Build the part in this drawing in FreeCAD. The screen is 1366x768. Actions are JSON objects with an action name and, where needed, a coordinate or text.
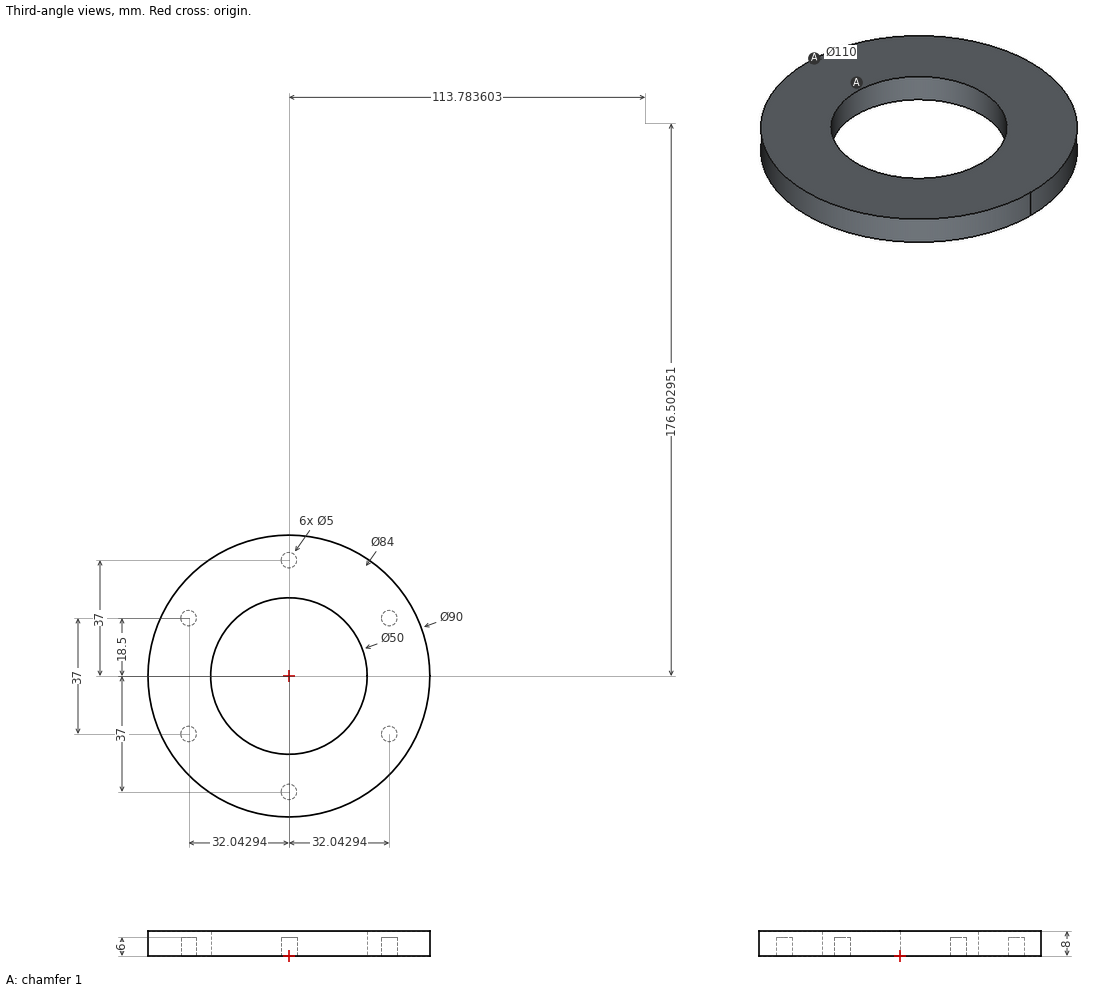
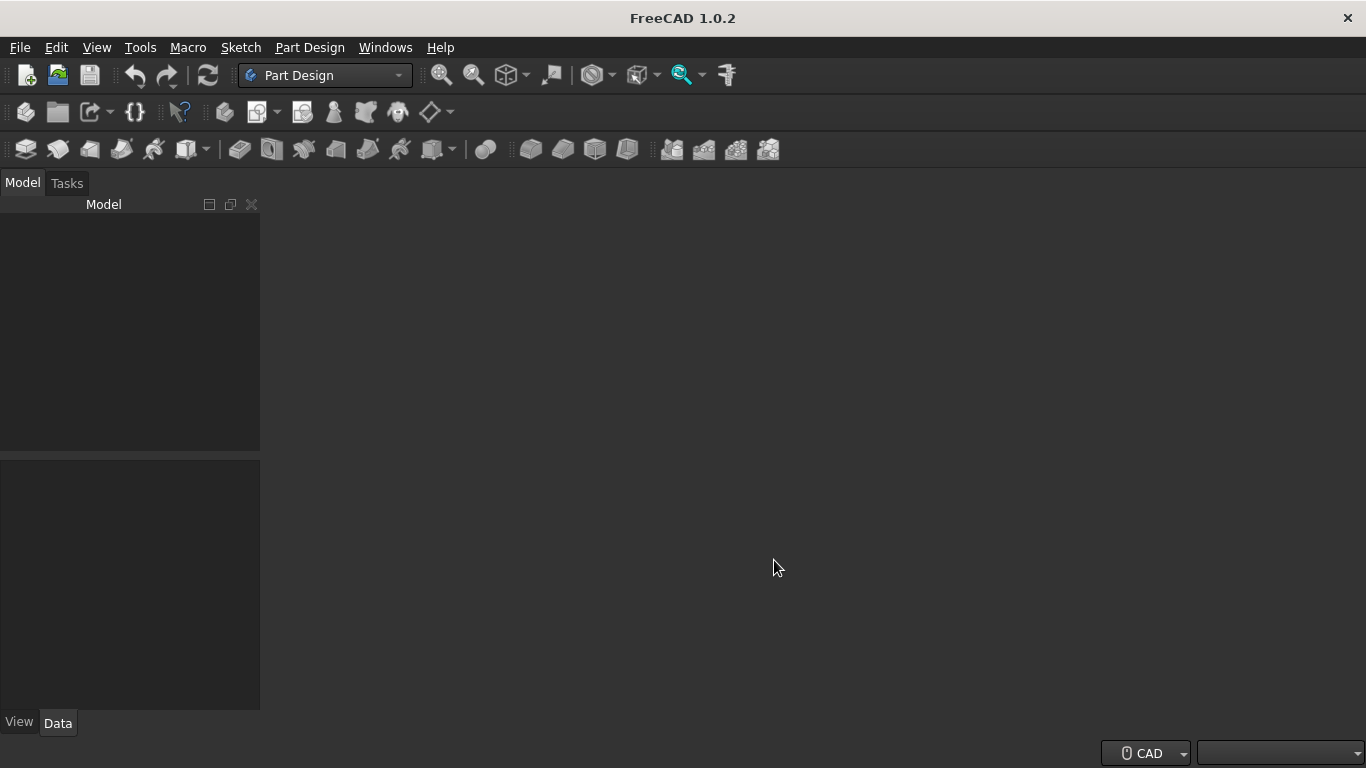
{"action": "left_click", "coordinate": [26, 76]}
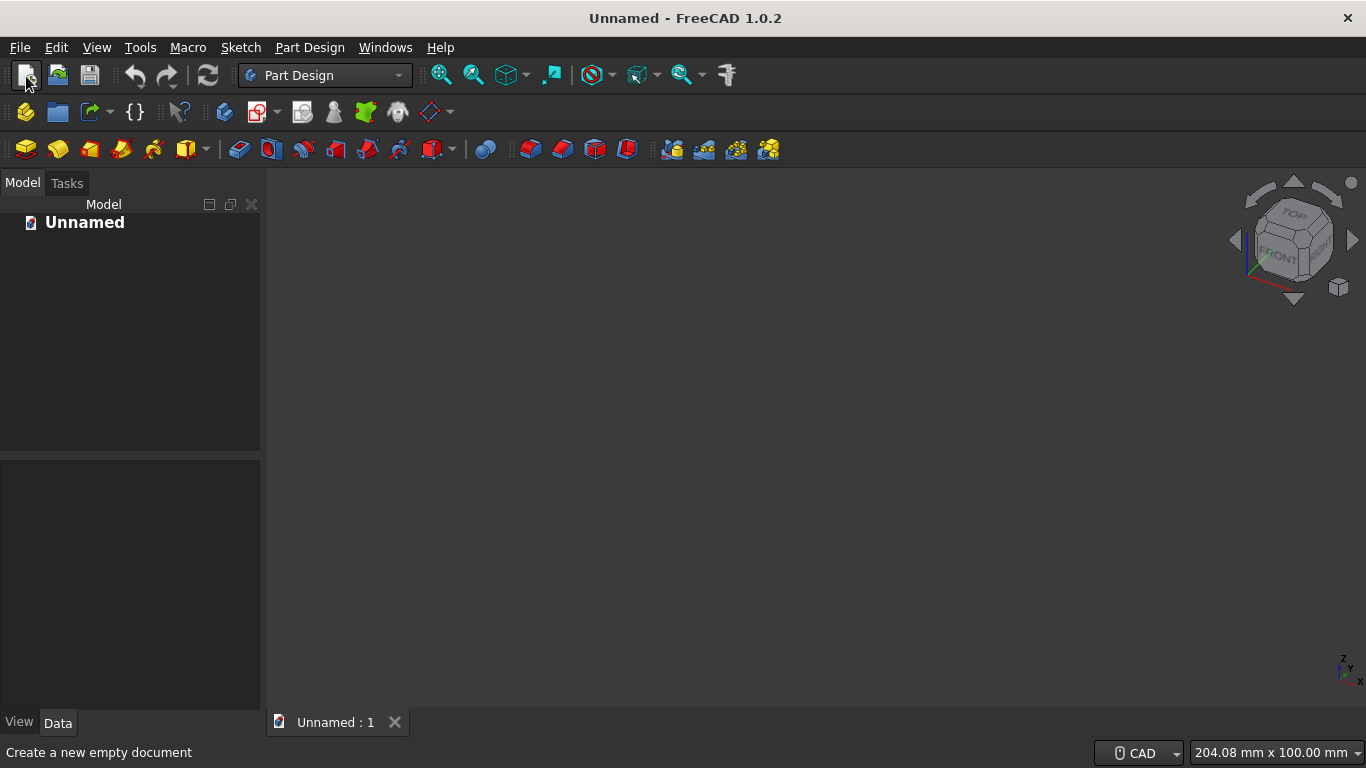
{"action": "left_click", "coordinate": [258, 112]}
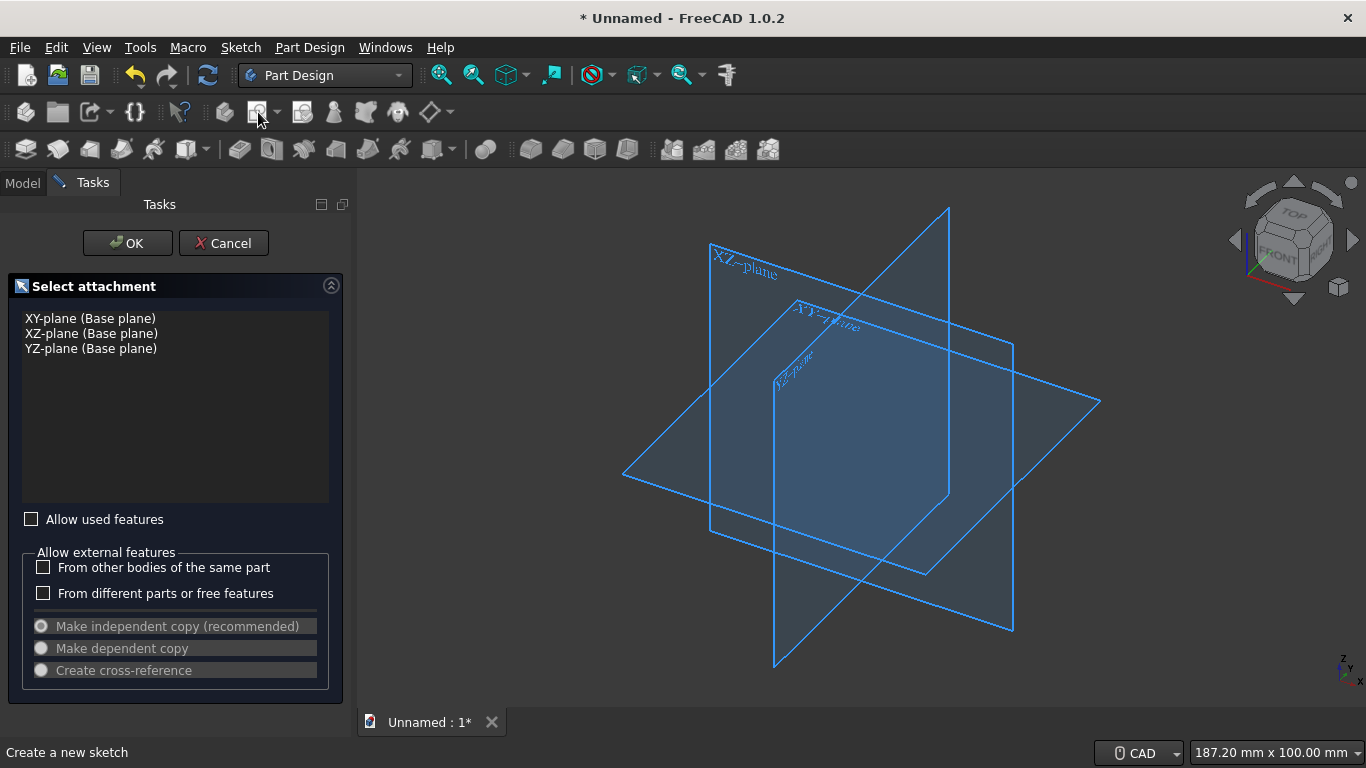
{"action": "left_click", "coordinate": [82, 318]}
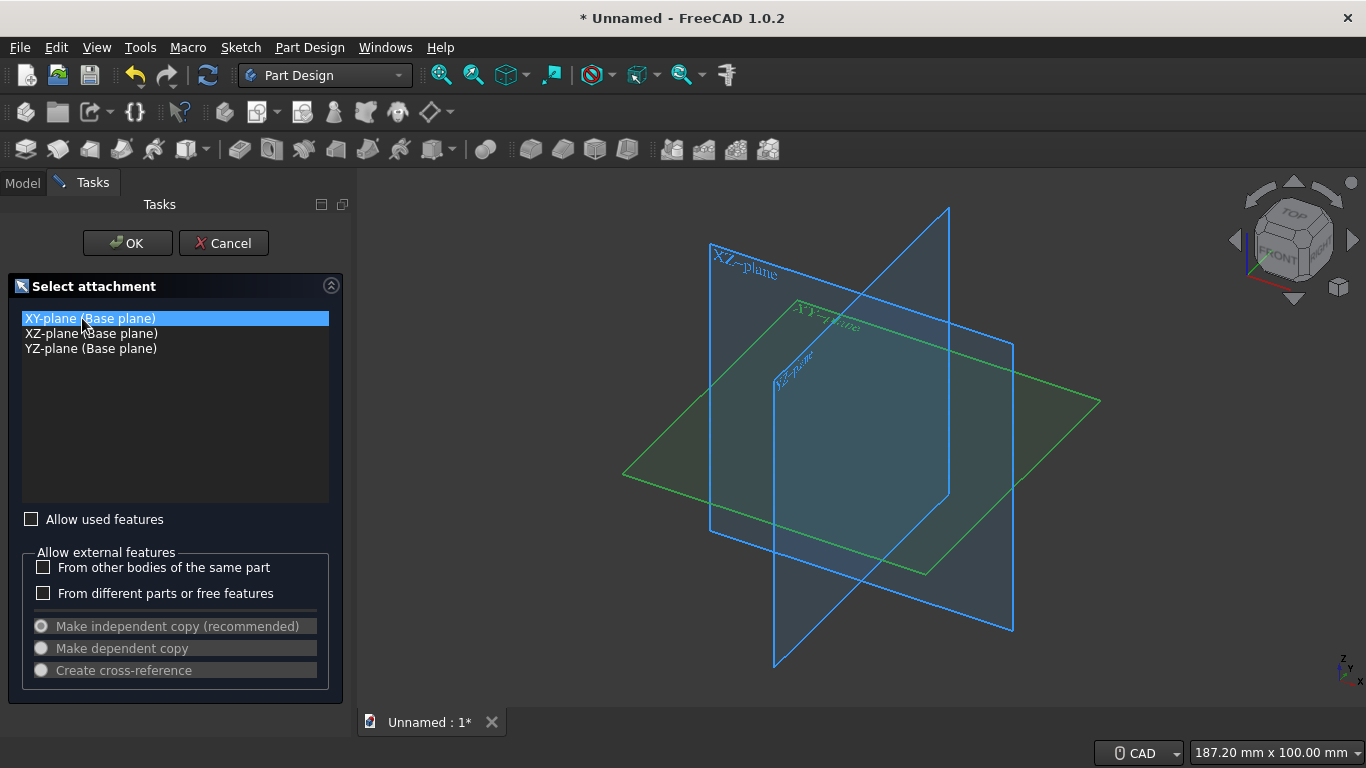
{"action": "left_click", "coordinate": [128, 243]}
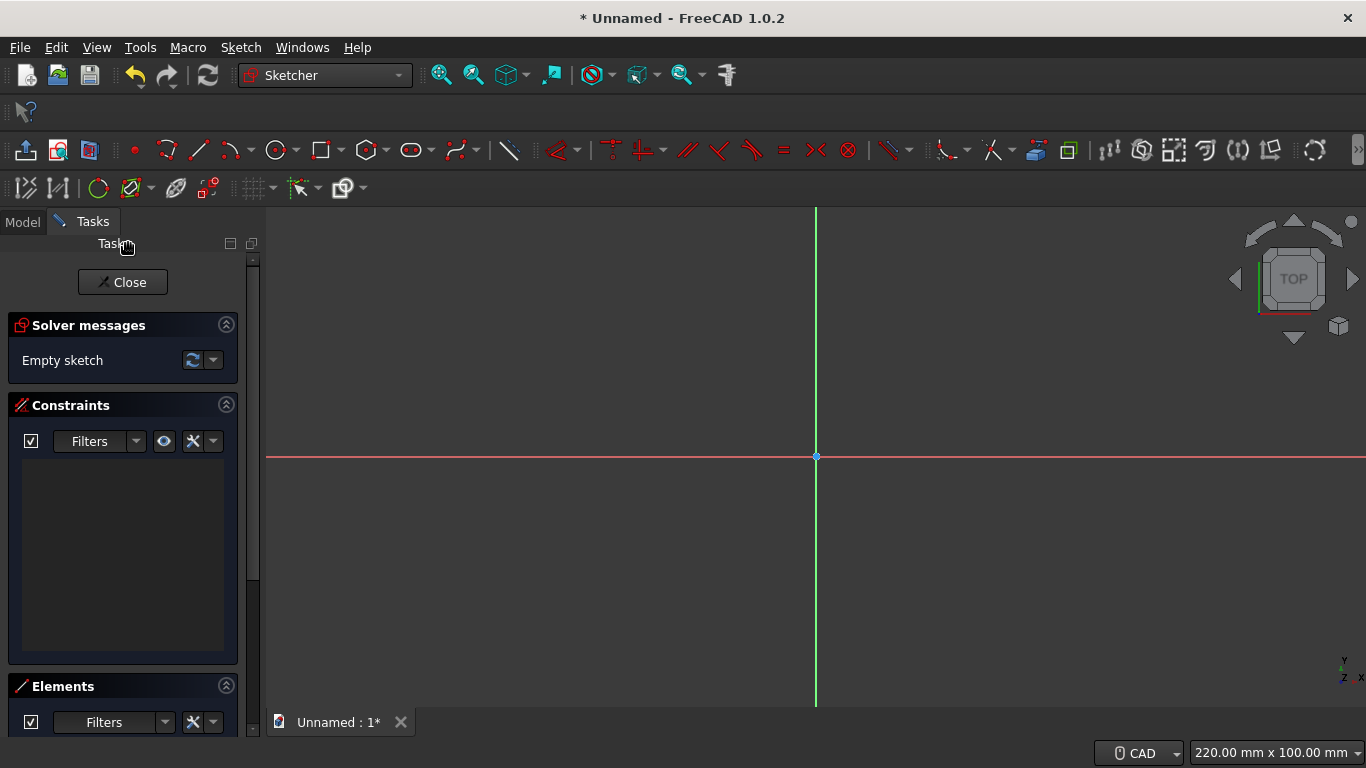
{"action": "scroll", "coordinate": [608, 457], "scroll_direction": "down", "scroll_amount": 2}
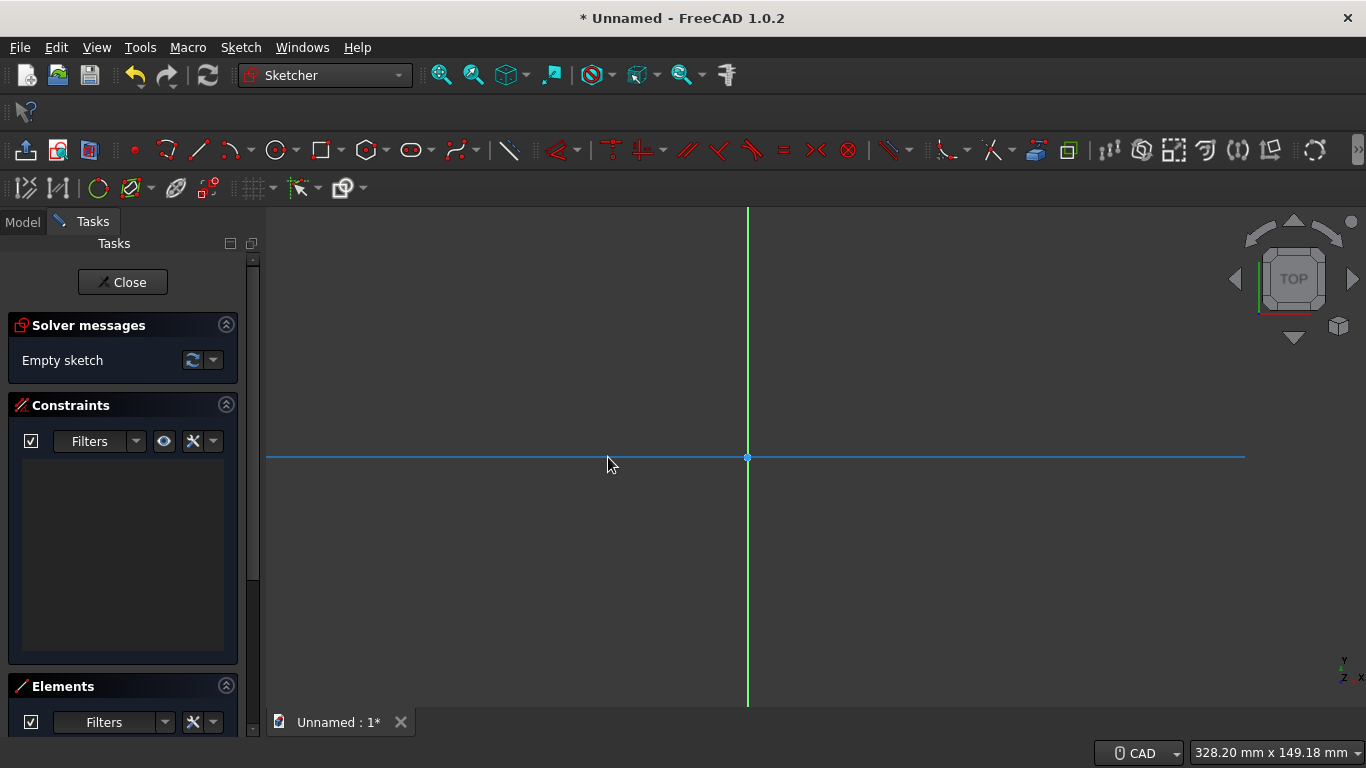
{"action": "key", "text": "g c"}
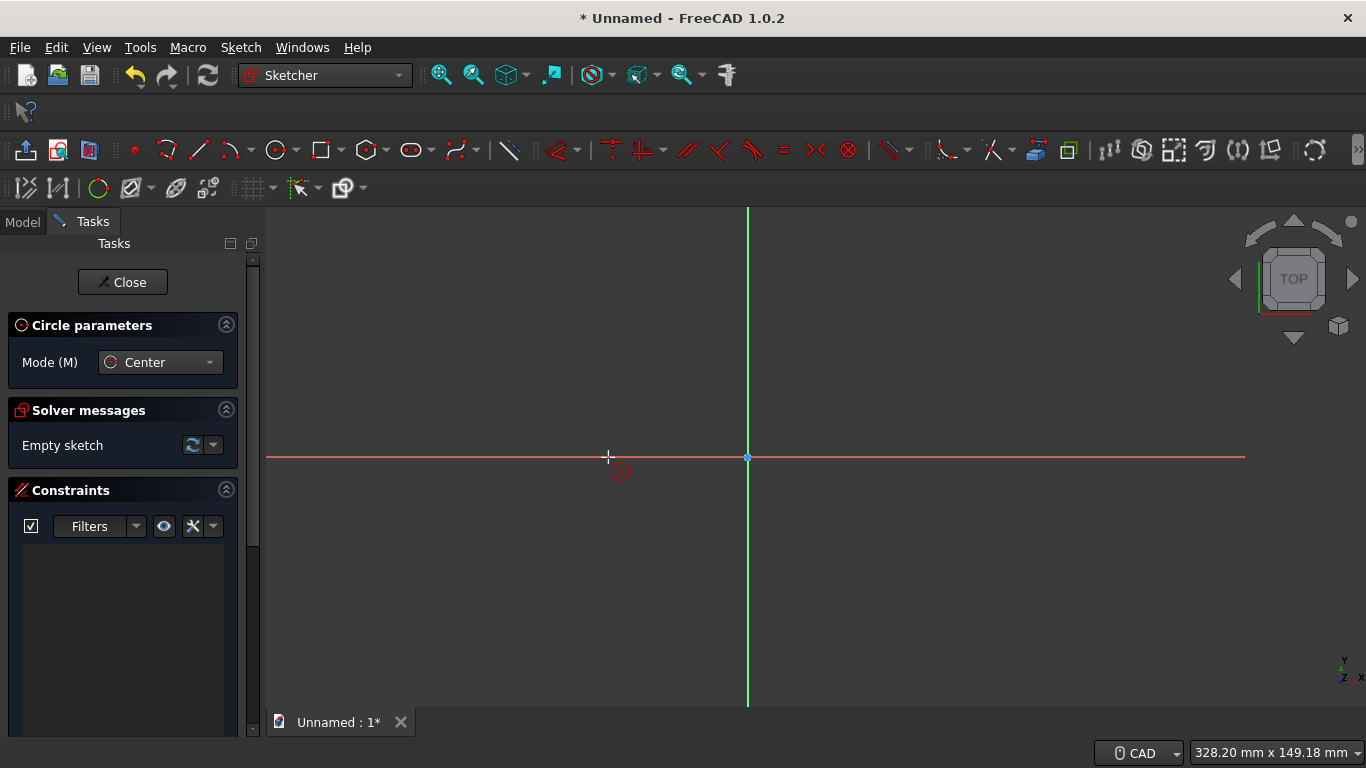
{"action": "left_click", "coordinate": [748, 457]}
{"action": "mouse_move", "coordinate": [854, 351]}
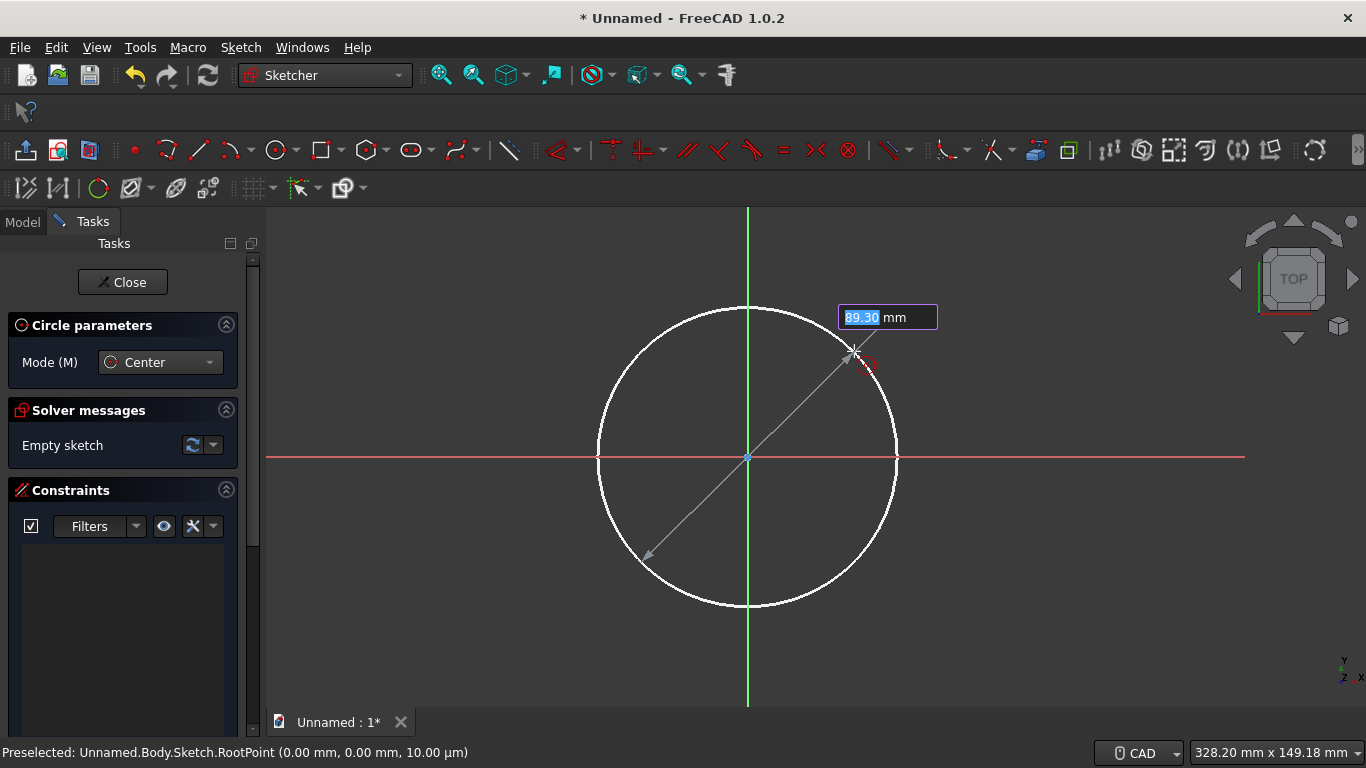
{"action": "type", "text": "90"}
{"action": "key", "text": "Return"}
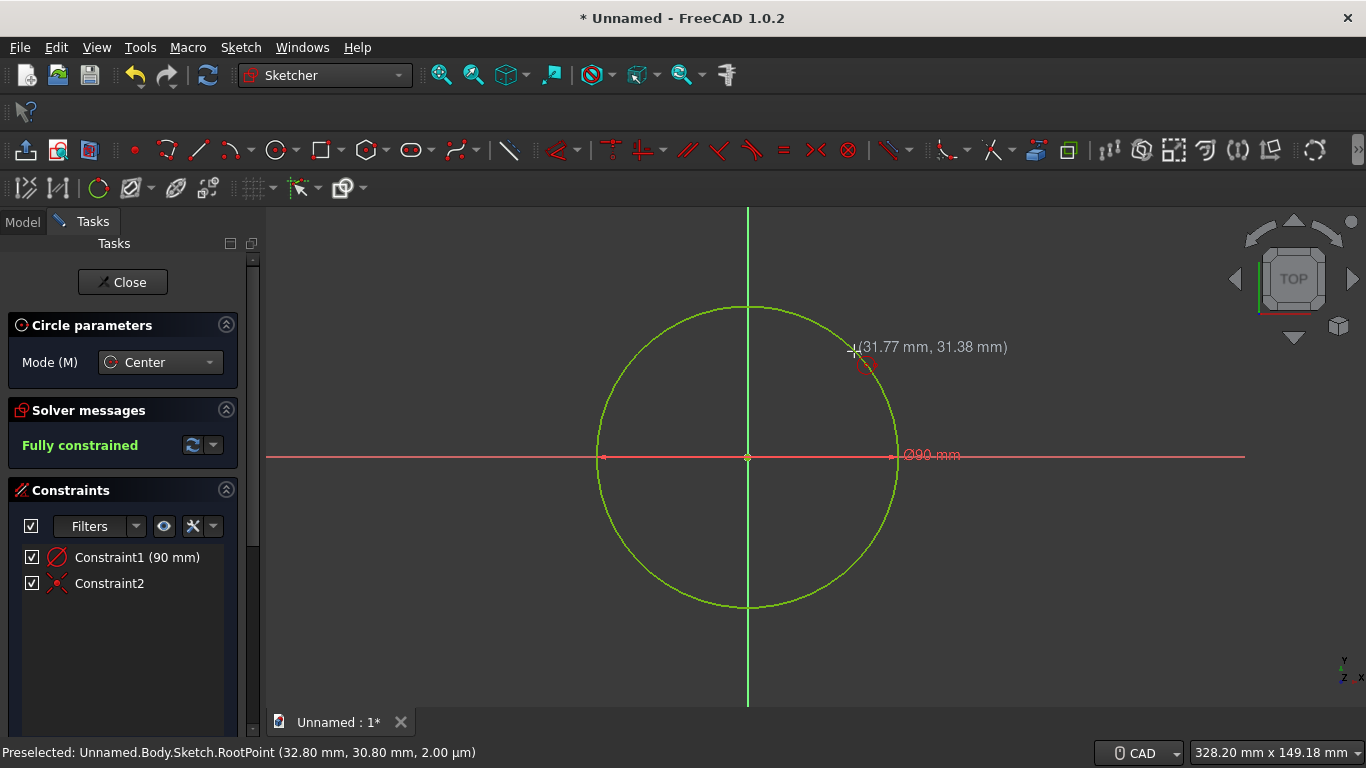
{"action": "left_click", "coordinate": [748, 457]}
{"action": "mouse_move", "coordinate": [807, 398]}